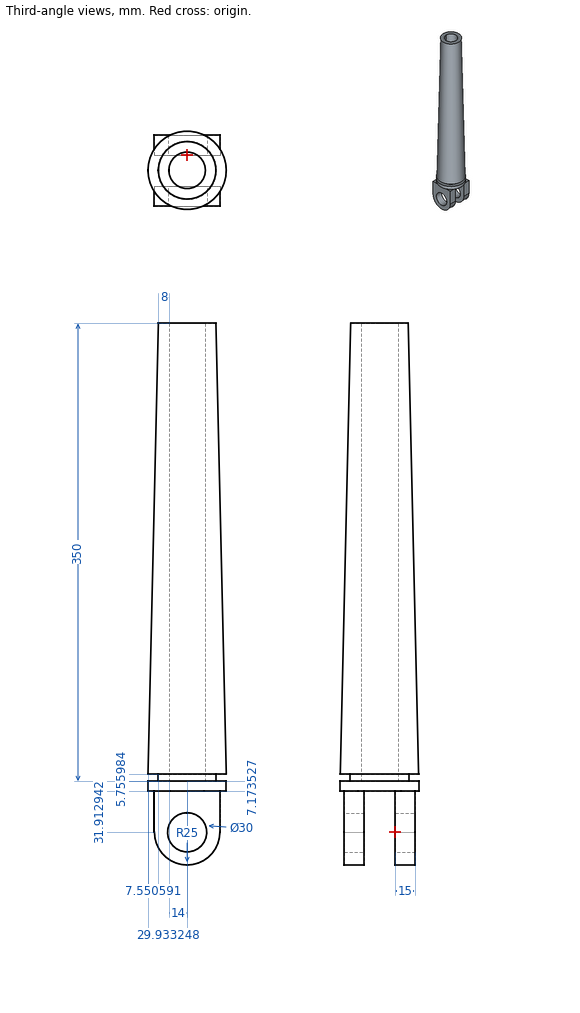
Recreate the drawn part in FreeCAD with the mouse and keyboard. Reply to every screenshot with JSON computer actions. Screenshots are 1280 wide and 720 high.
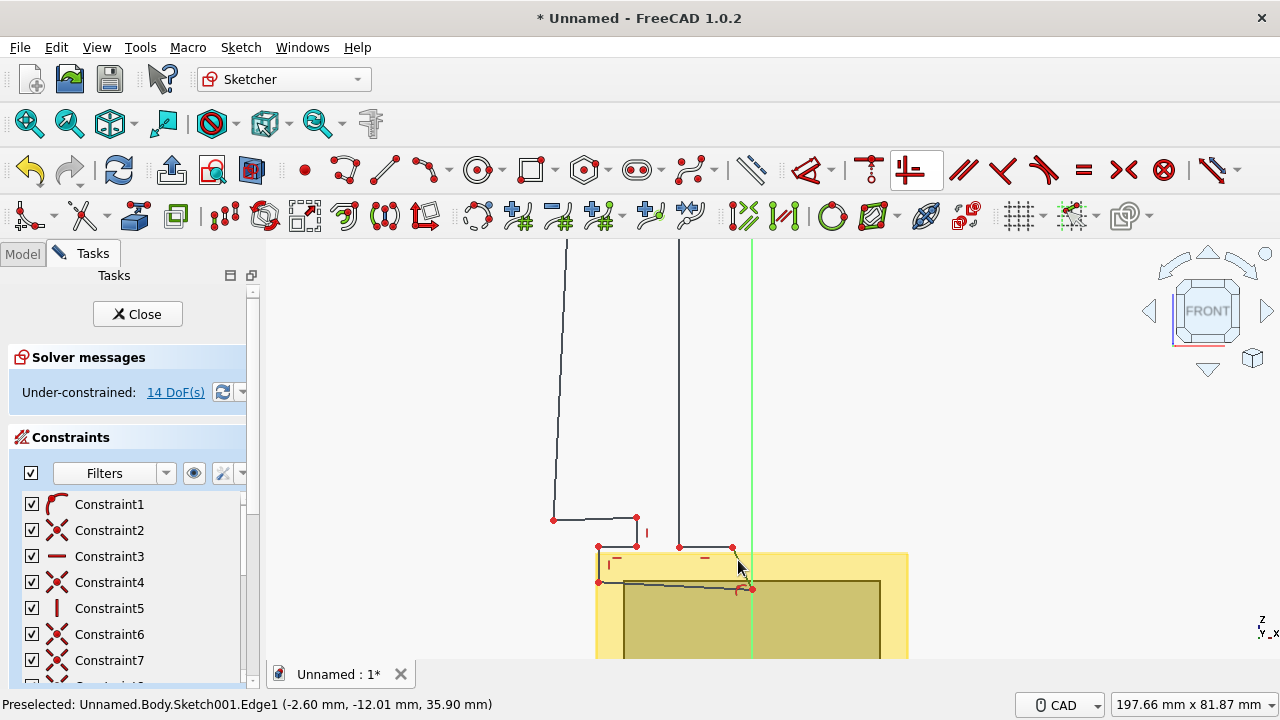
{"action": "key", "text": "v"}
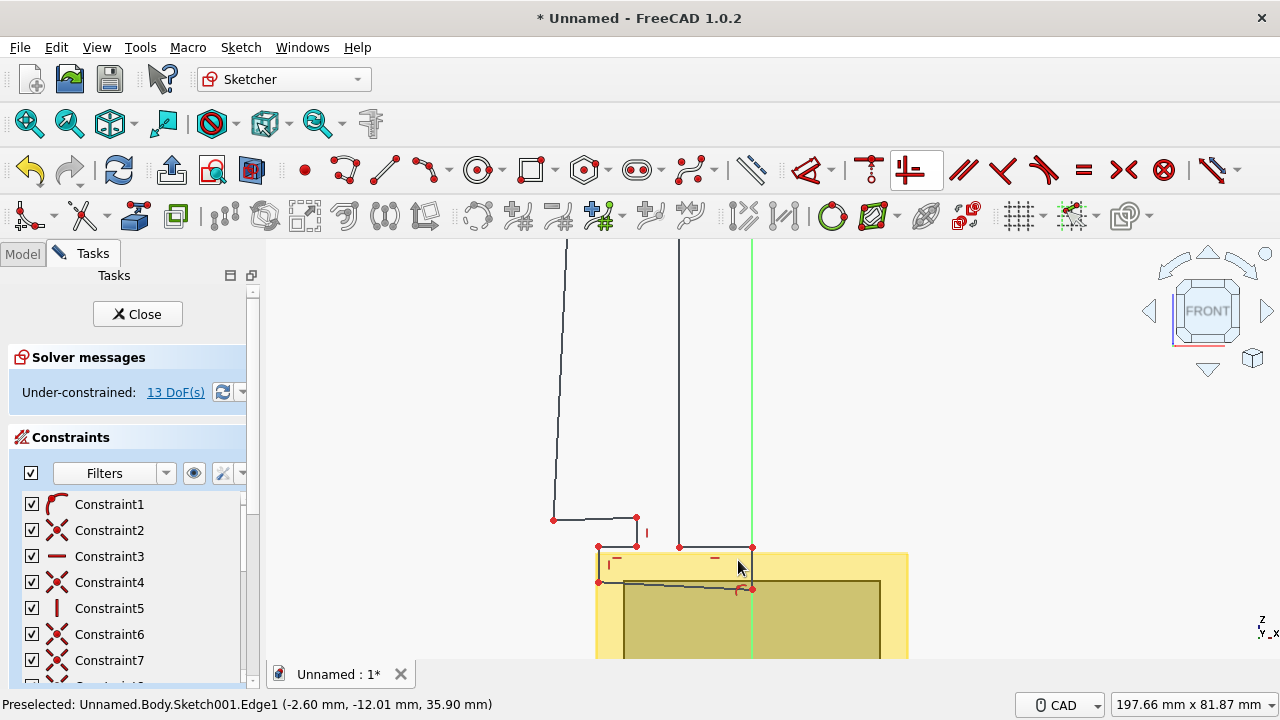
{"action": "scroll", "coordinate": [709, 559], "scroll_direction": "down", "scroll_amount": 10}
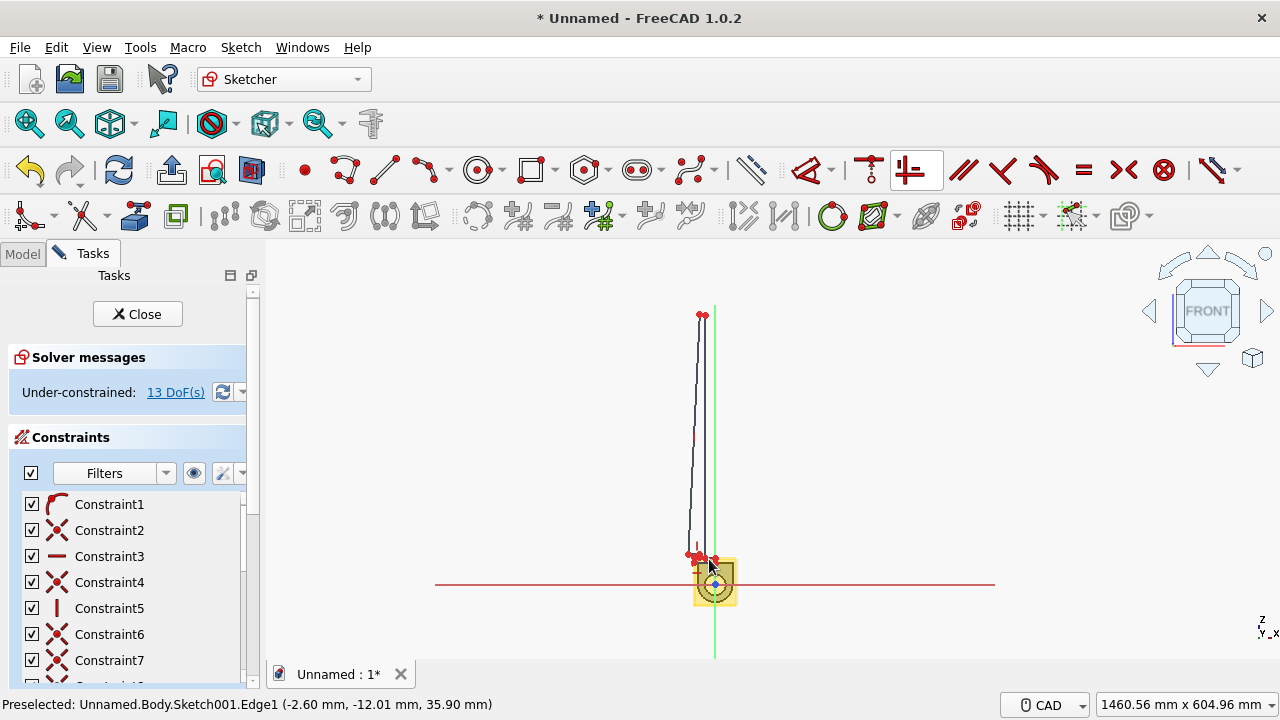
{"action": "scroll", "coordinate": [704, 315], "scroll_direction": "up", "scroll_amount": 11}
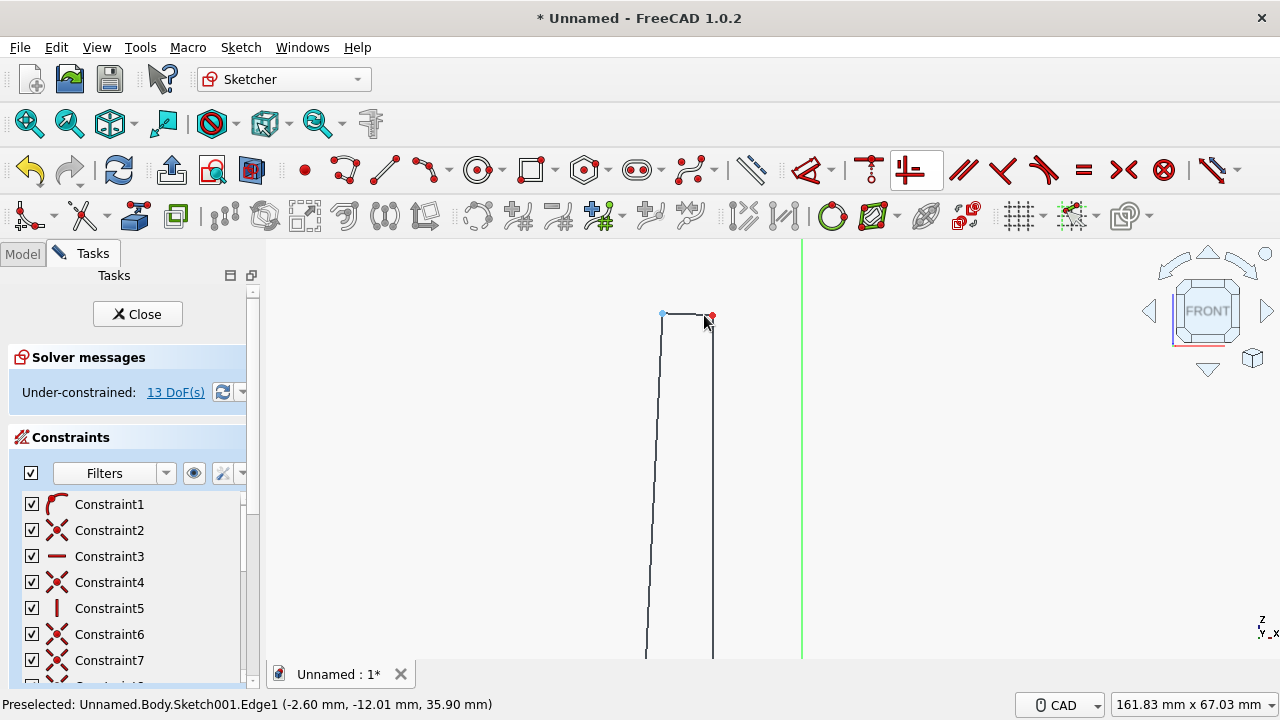
{"action": "left_click", "coordinate": [698, 315]}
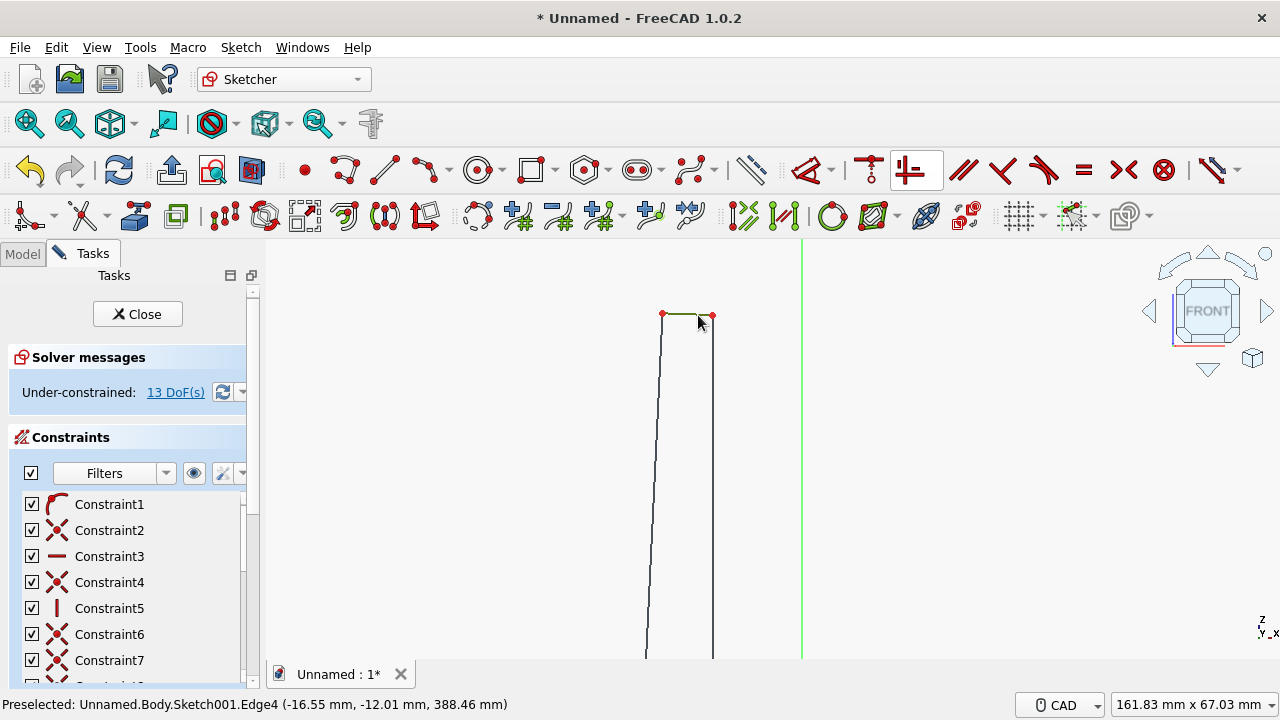
{"action": "key", "text": "h"}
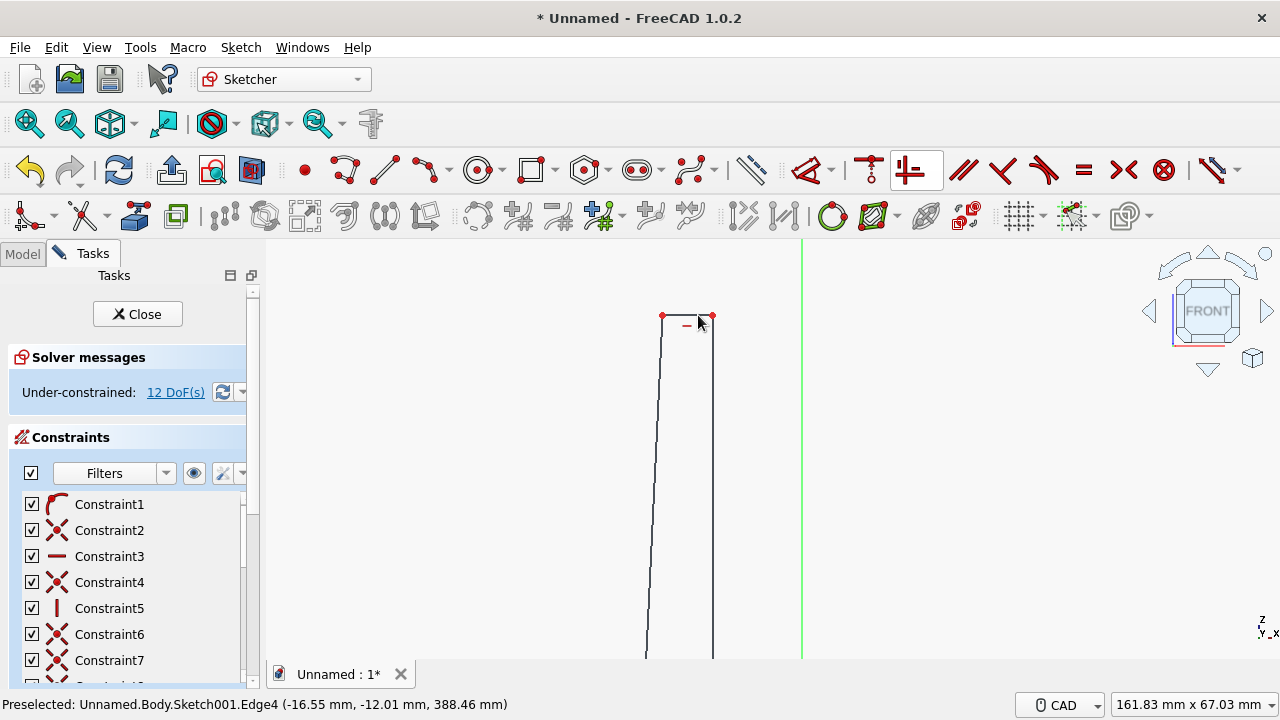
{"action": "scroll", "coordinate": [704, 314], "scroll_direction": "down", "scroll_amount": 11}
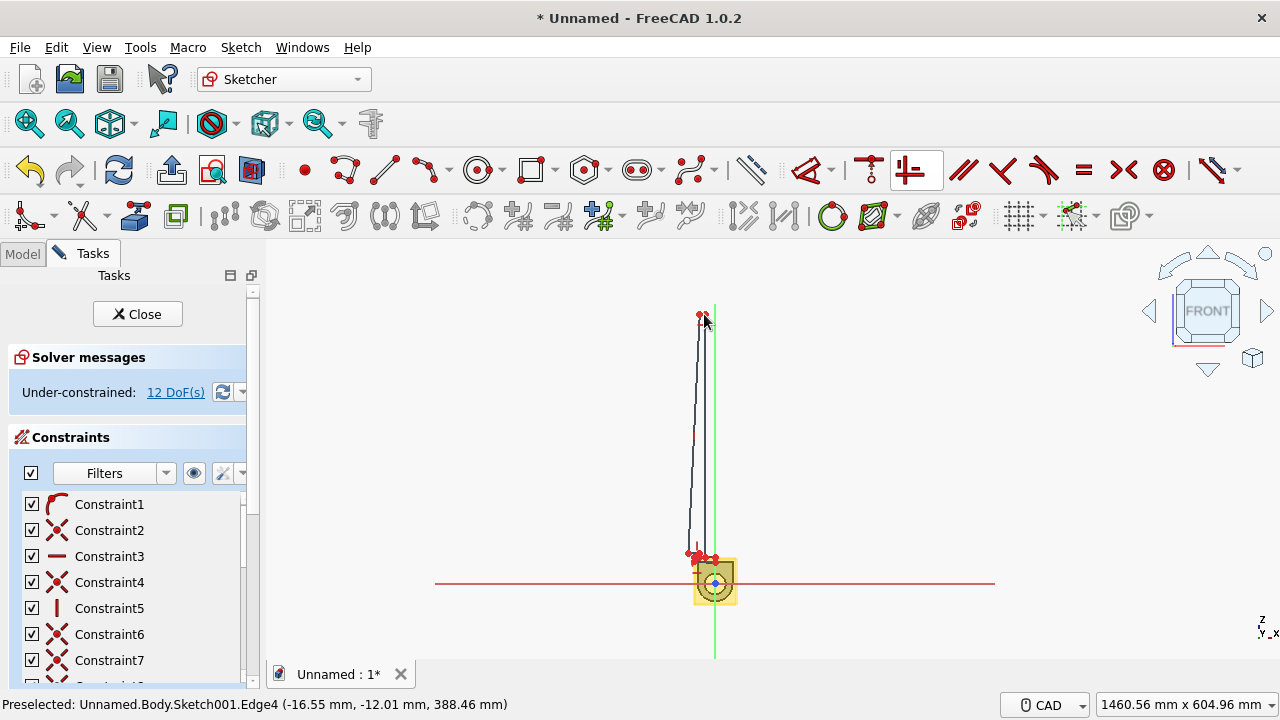
{"action": "scroll", "coordinate": [692, 553], "scroll_direction": "up", "scroll_amount": 8}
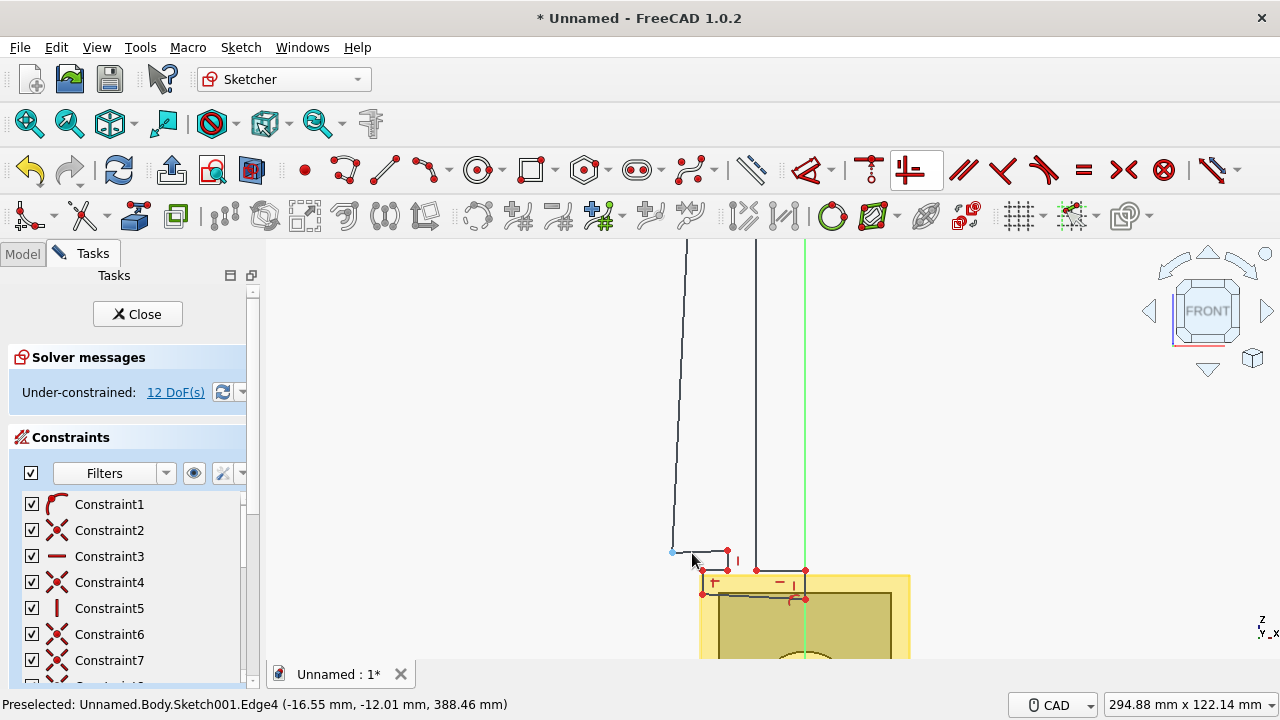
{"action": "left_click", "coordinate": [689, 552]}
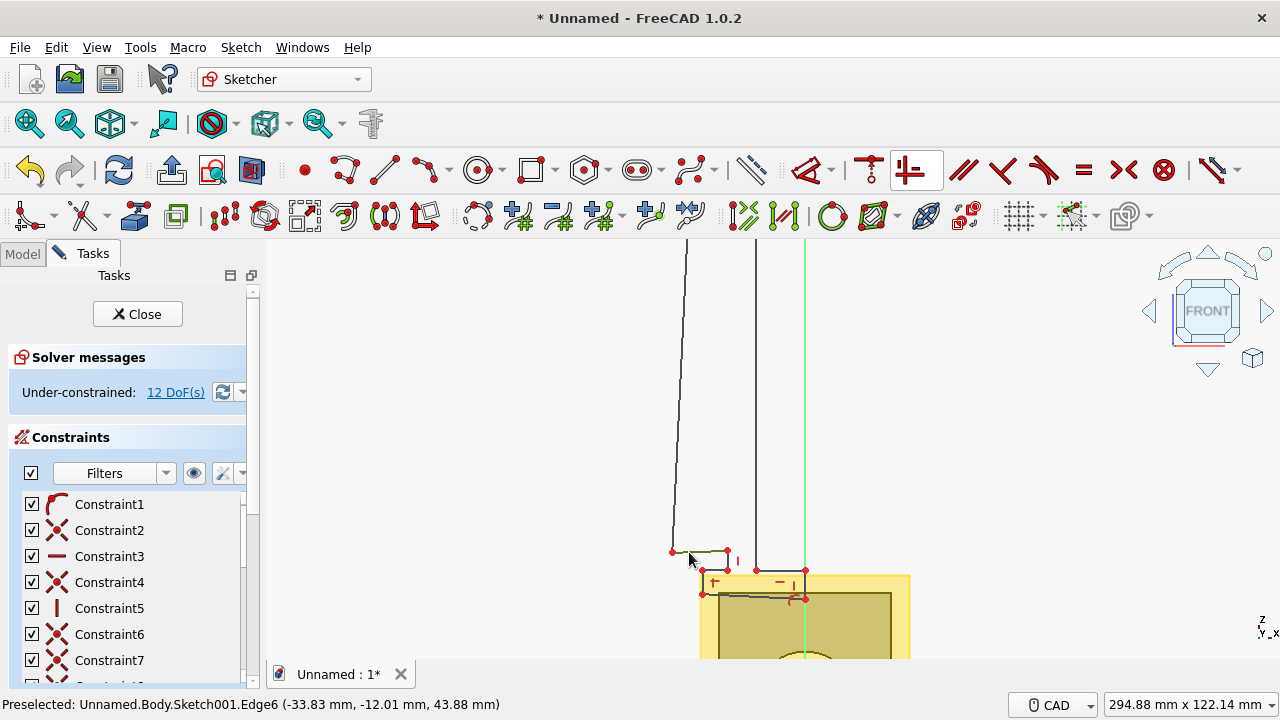
{"action": "left_click", "coordinate": [938, 170]}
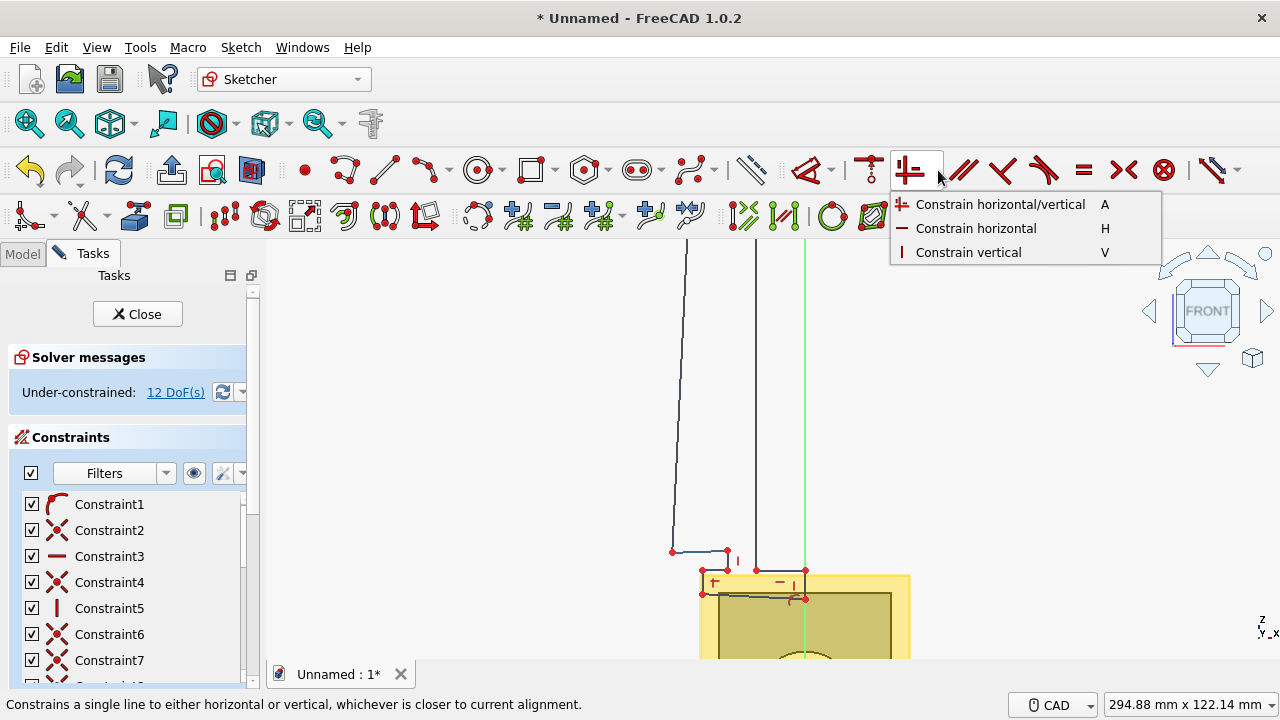
{"action": "left_click", "coordinate": [1026, 228]}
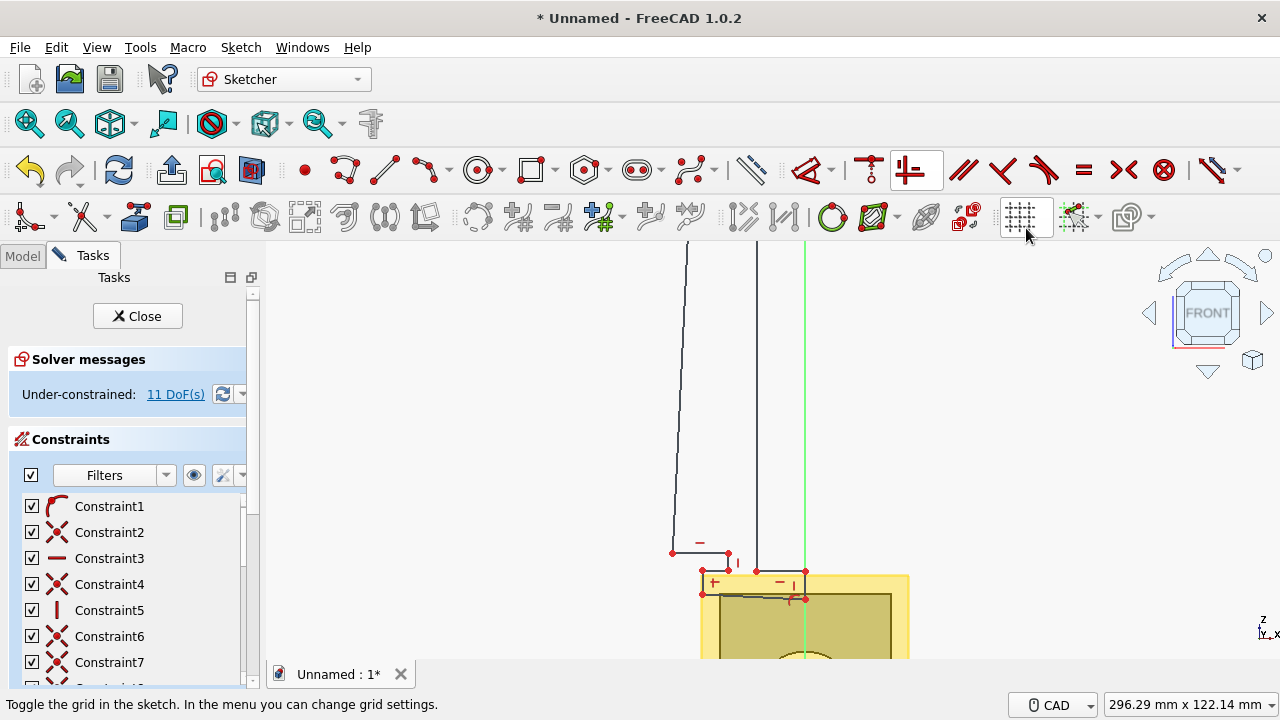
{"action": "left_click", "coordinate": [734, 596]}